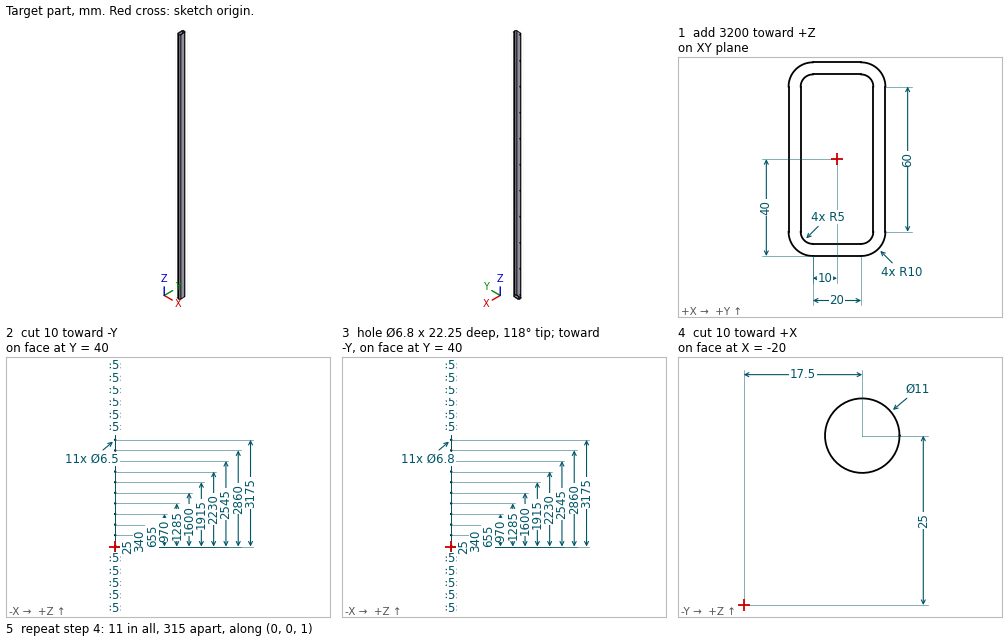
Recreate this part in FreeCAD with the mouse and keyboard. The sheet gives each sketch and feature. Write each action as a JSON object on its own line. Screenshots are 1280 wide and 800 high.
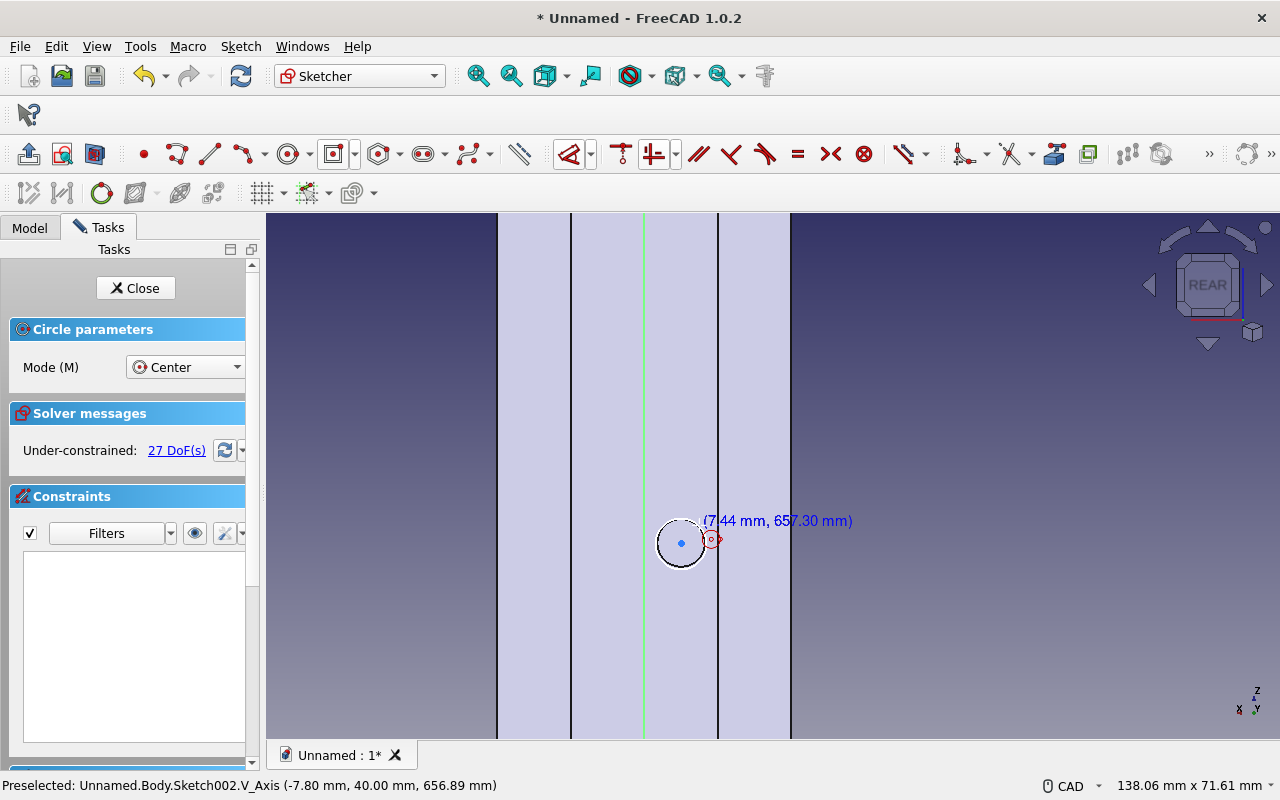
{"action": "scroll", "coordinate": [704, 476], "scroll_direction": "down", "scroll_amount": 15}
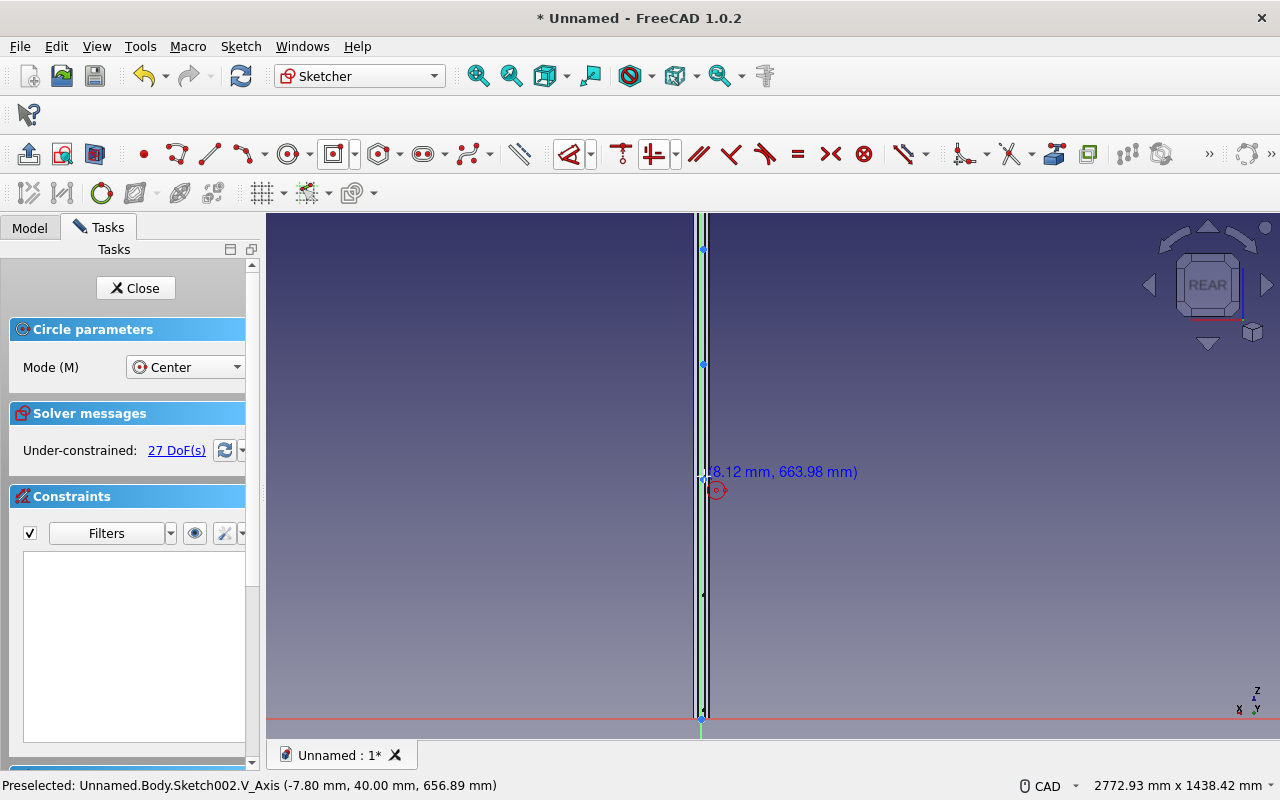
{"action": "scroll", "coordinate": [705, 622], "scroll_direction": "down", "scroll_amount": 6}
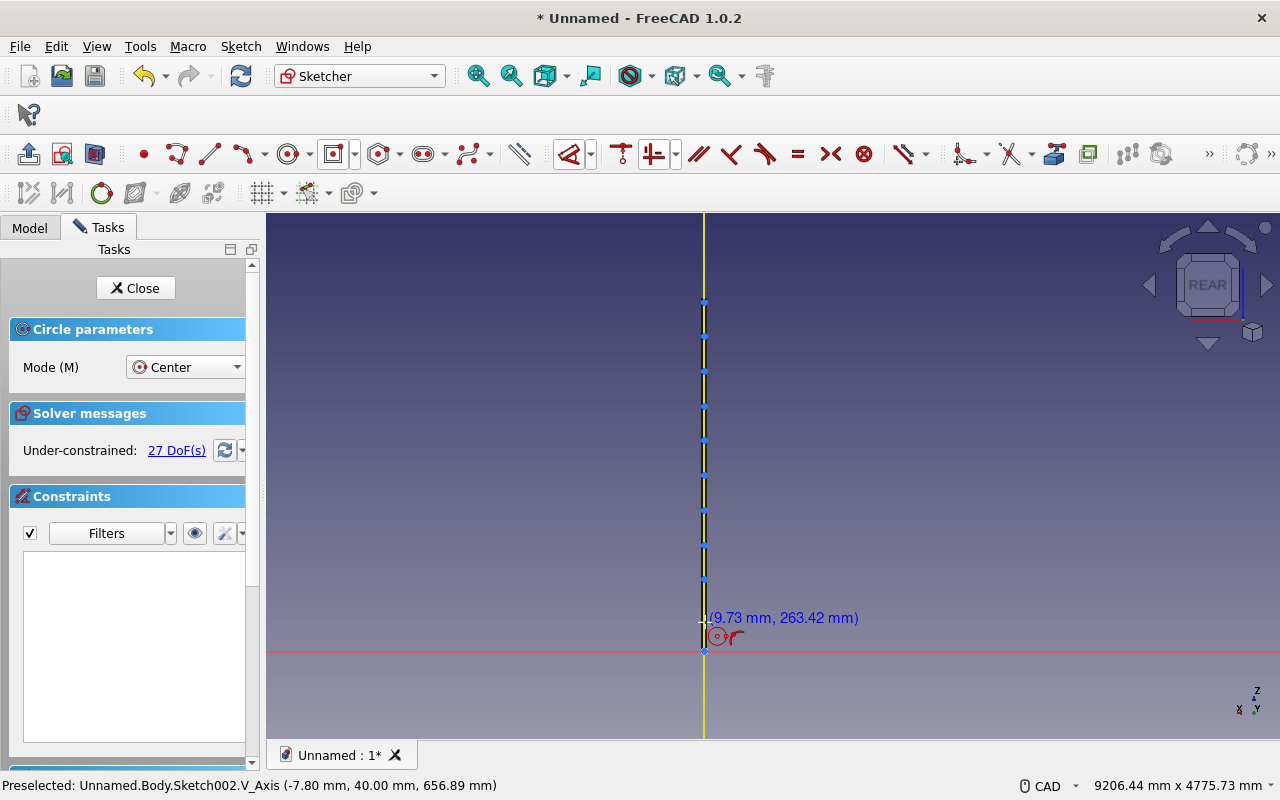
{"action": "scroll", "coordinate": [705, 614], "scroll_direction": "up", "scroll_amount": 21}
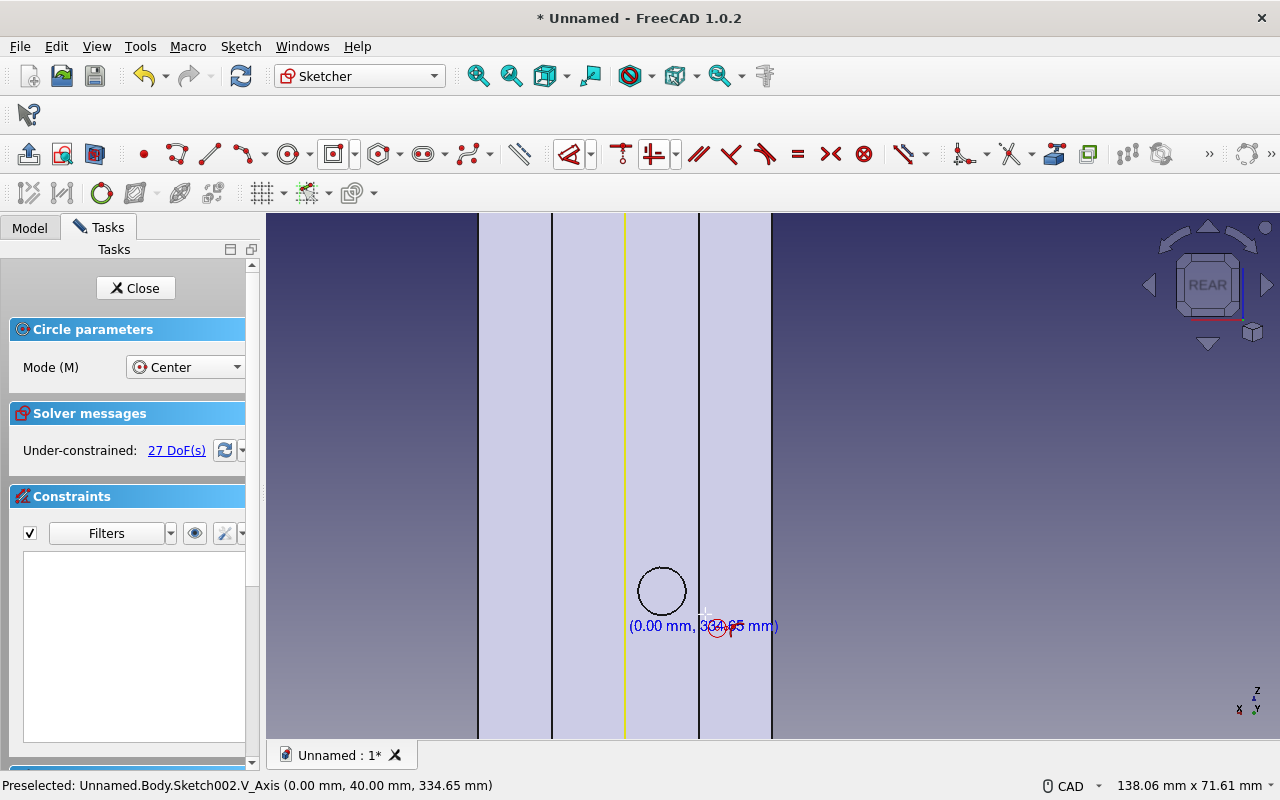
{"action": "left_click", "coordinate": [662, 591]}
{"action": "left_click", "coordinate": [680, 574]}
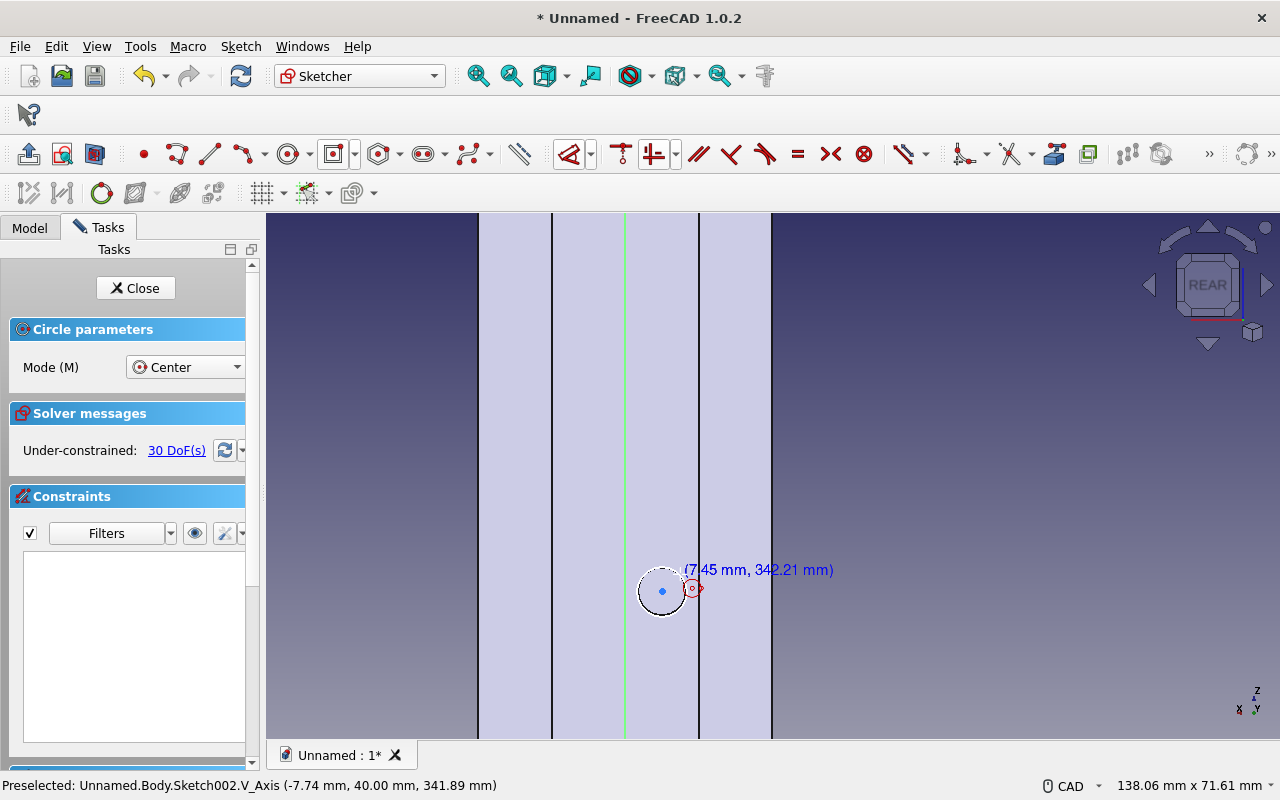
{"action": "scroll", "coordinate": [704, 476], "scroll_direction": "down", "scroll_amount": 15}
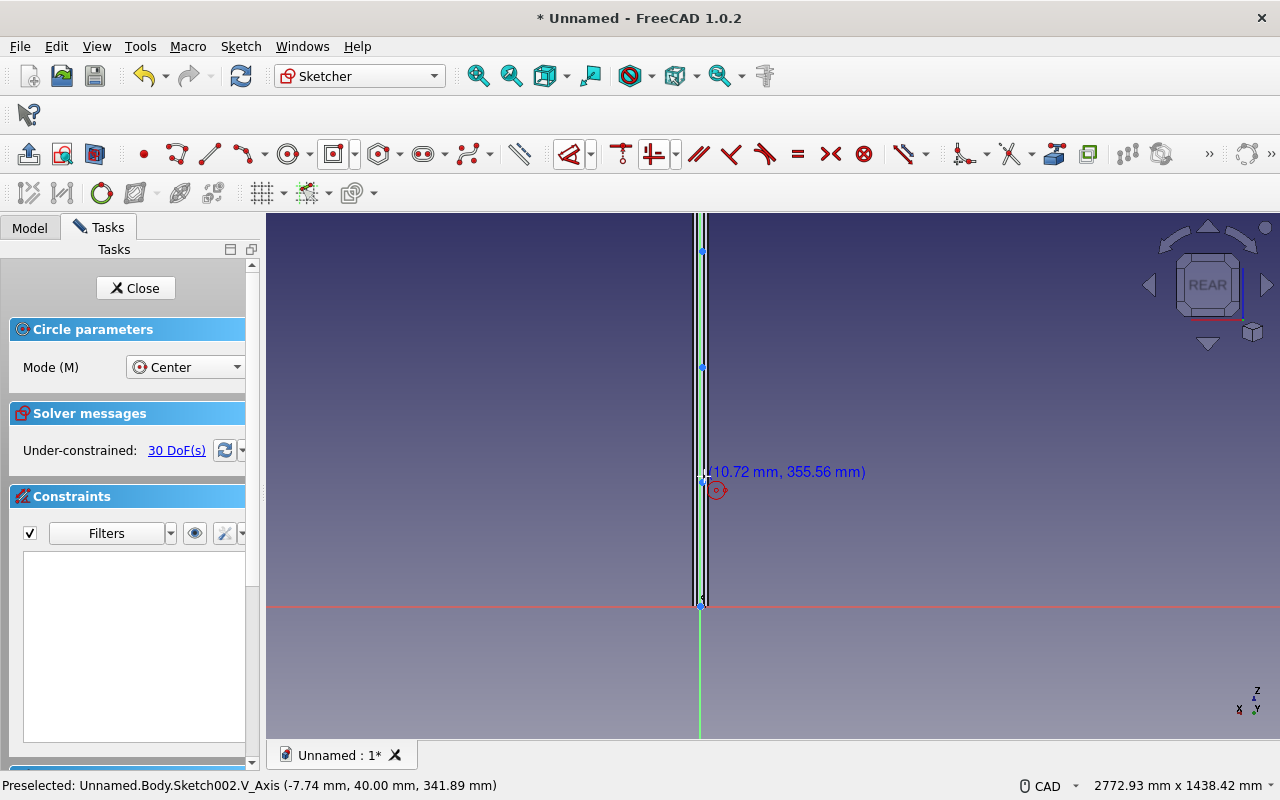
{"action": "scroll", "coordinate": [706, 670], "scroll_direction": "down", "scroll_amount": 6}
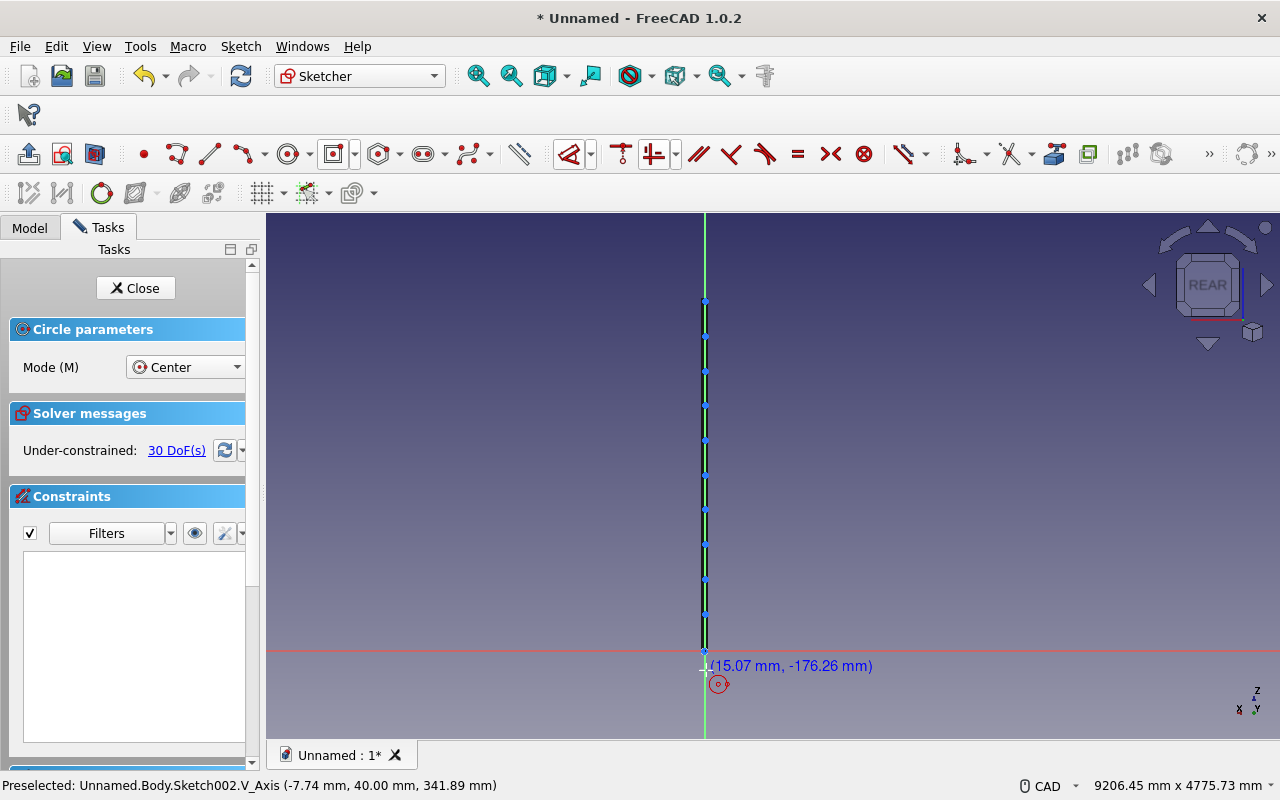
{"action": "scroll", "coordinate": [705, 649], "scroll_direction": "up", "scroll_amount": 21}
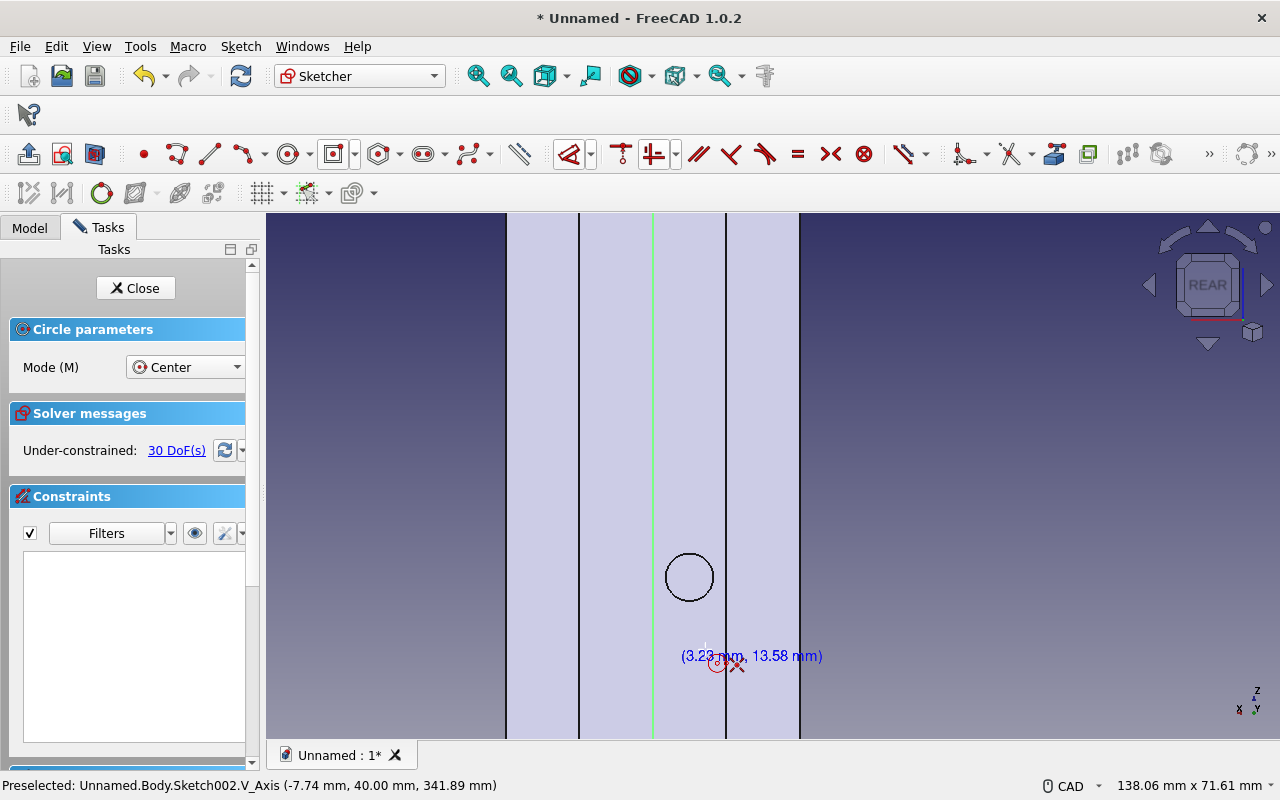
{"action": "left_click", "coordinate": [690, 577]}
{"action": "left_click", "coordinate": [707, 560]}
{"action": "key", "text": "Escape"}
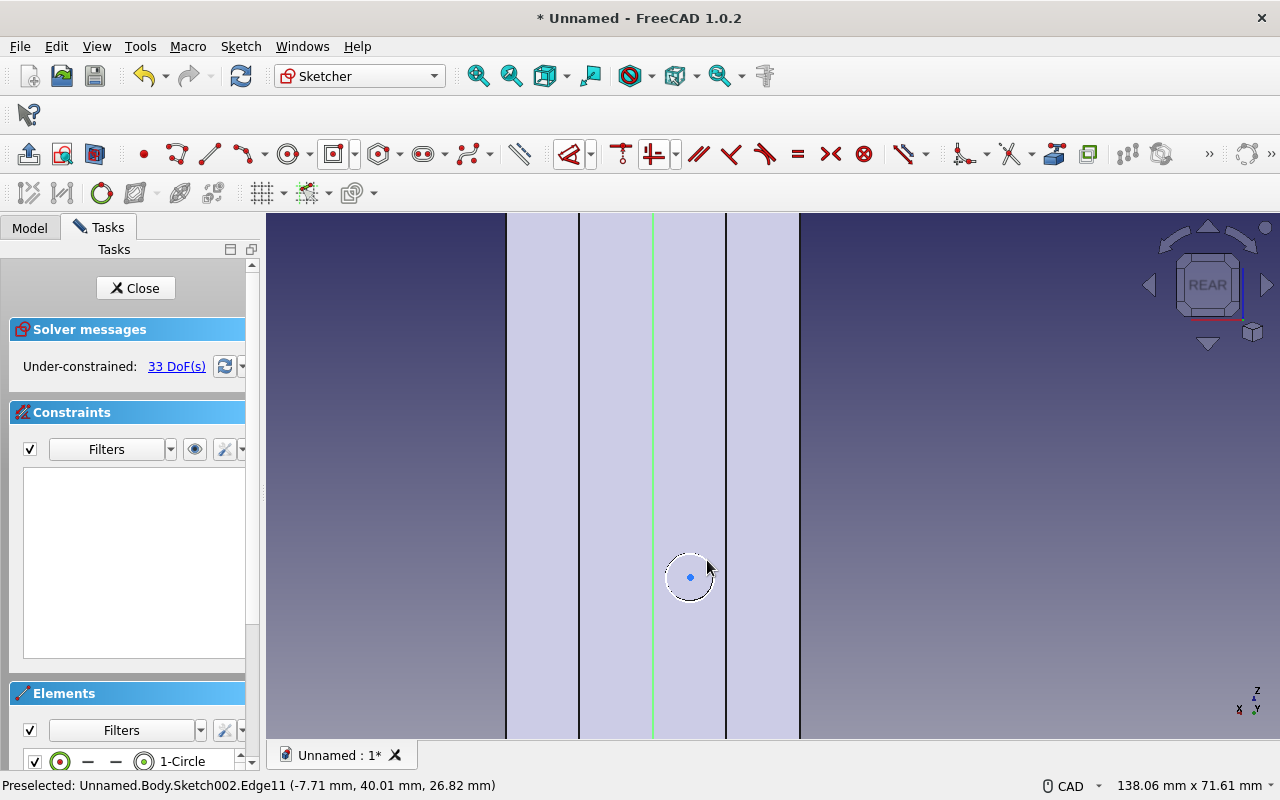
{"action": "scroll", "coordinate": [704, 476], "scroll_direction": "down", "scroll_amount": 15}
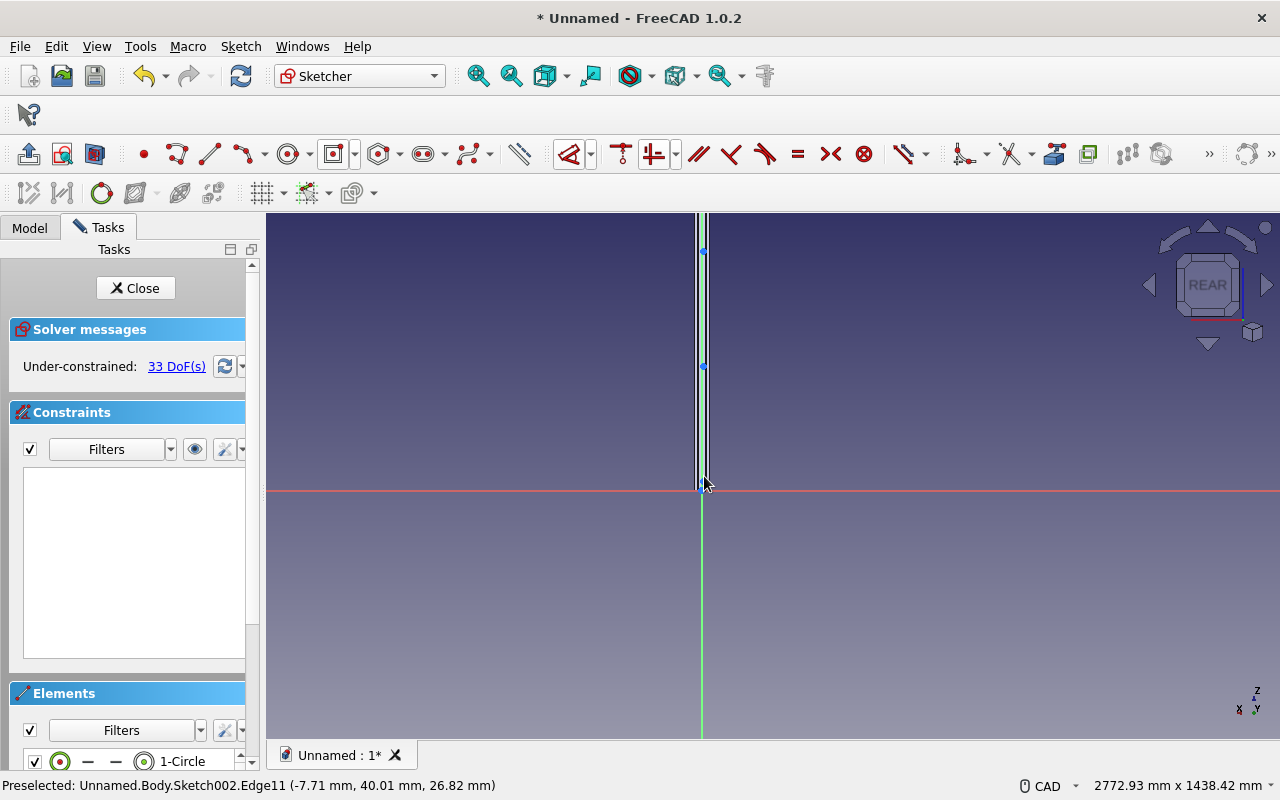
{"action": "scroll", "coordinate": [705, 711], "scroll_direction": "down", "scroll_amount": 6}